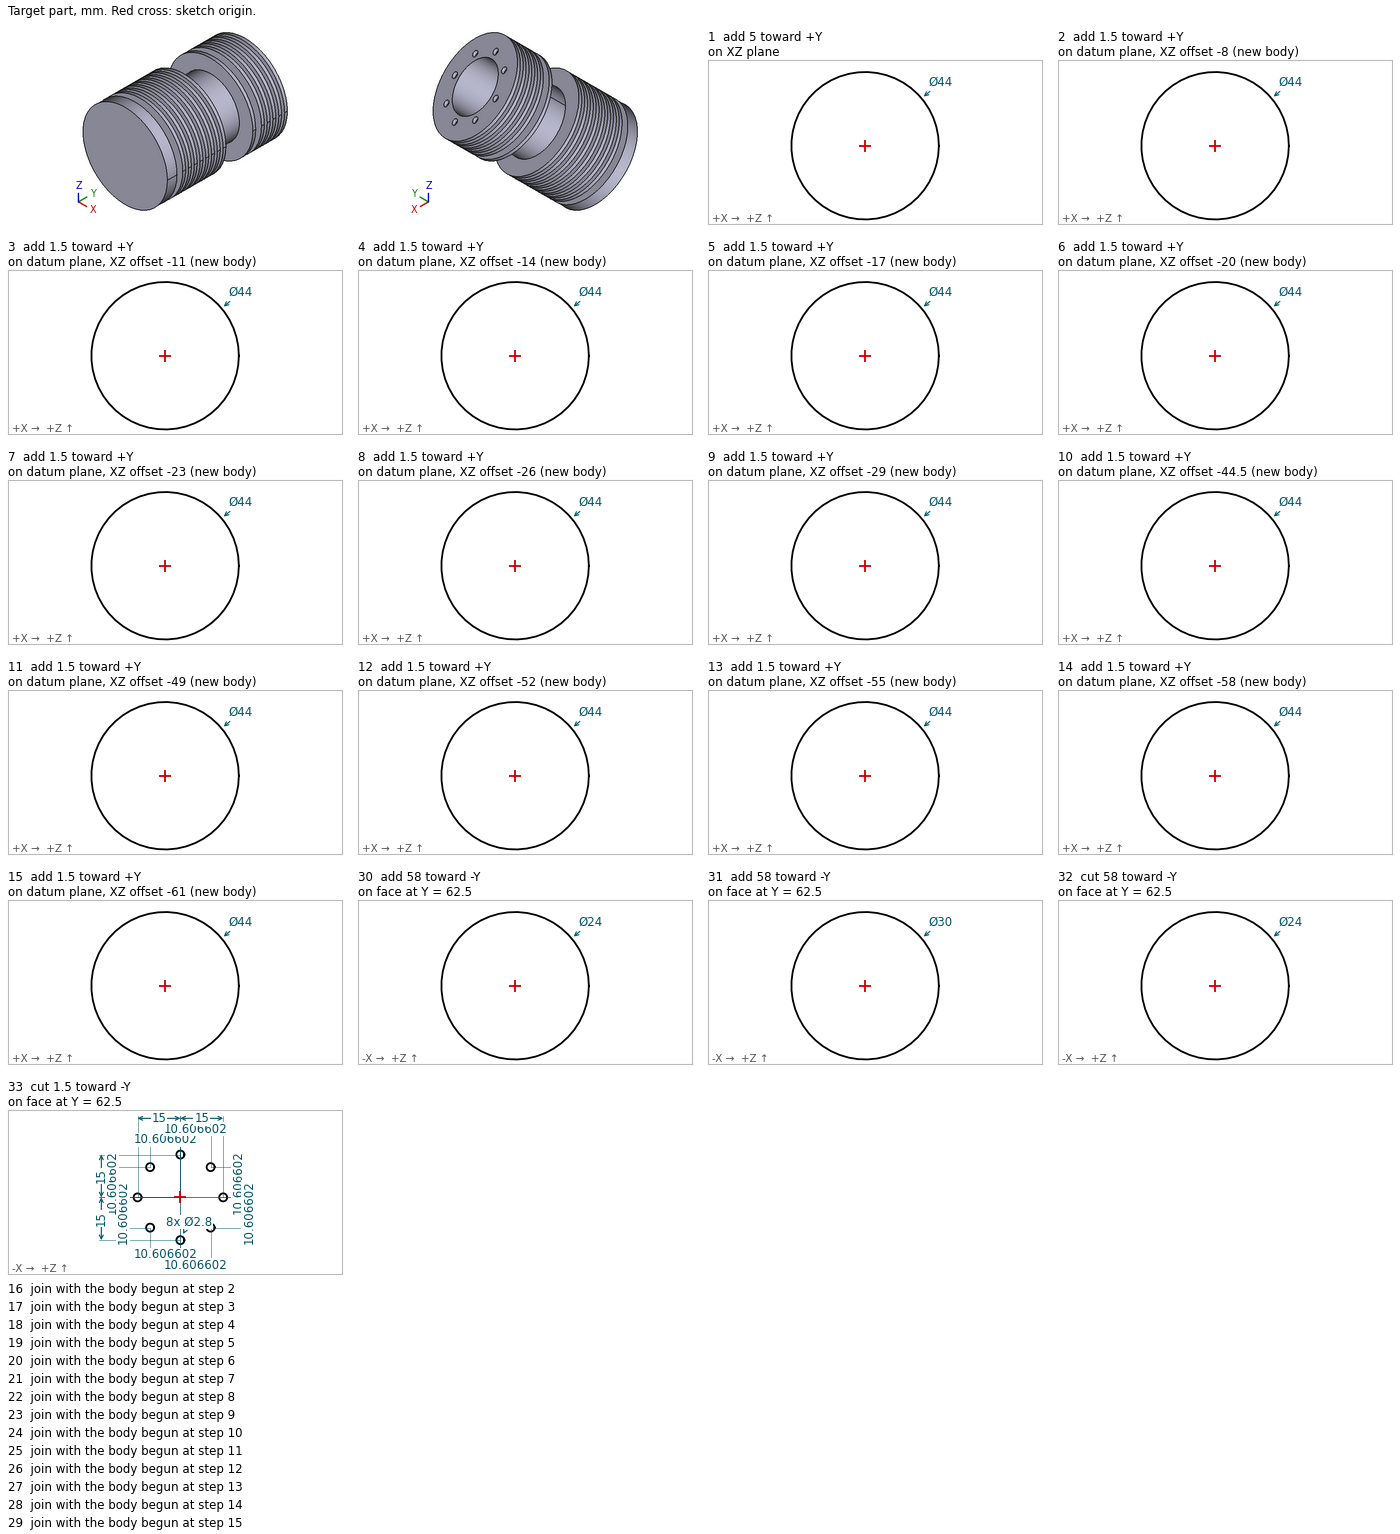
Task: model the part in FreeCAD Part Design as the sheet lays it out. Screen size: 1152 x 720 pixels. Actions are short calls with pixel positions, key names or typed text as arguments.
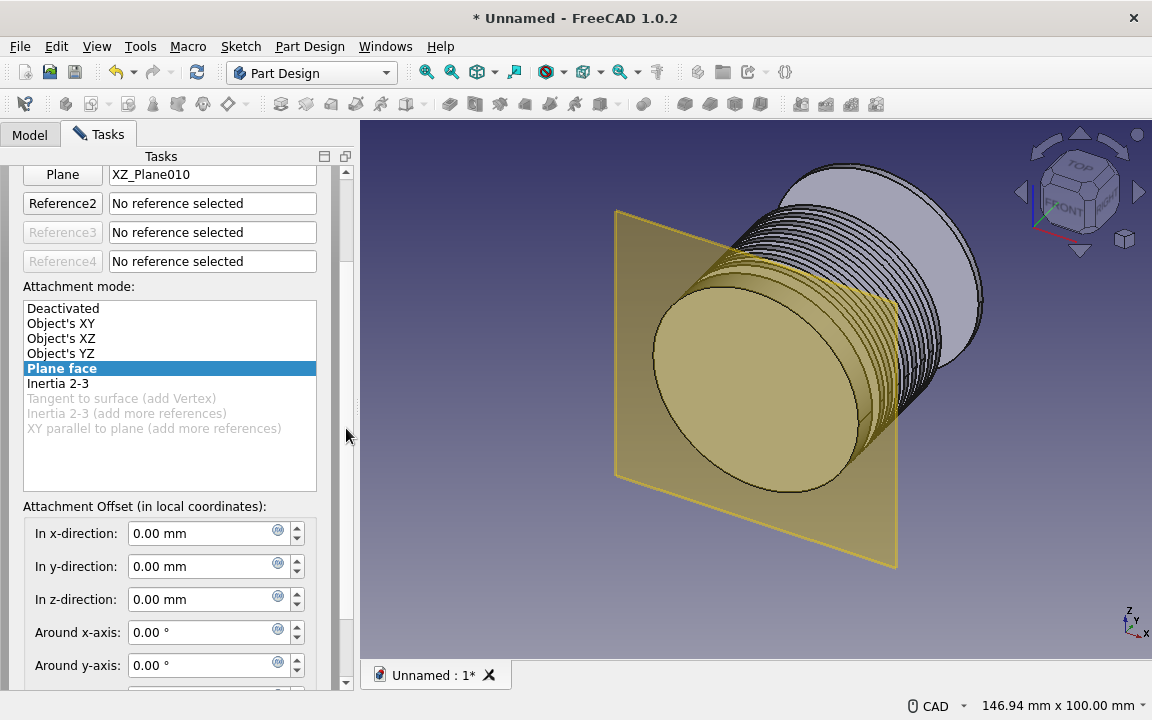
triple_click(210, 600)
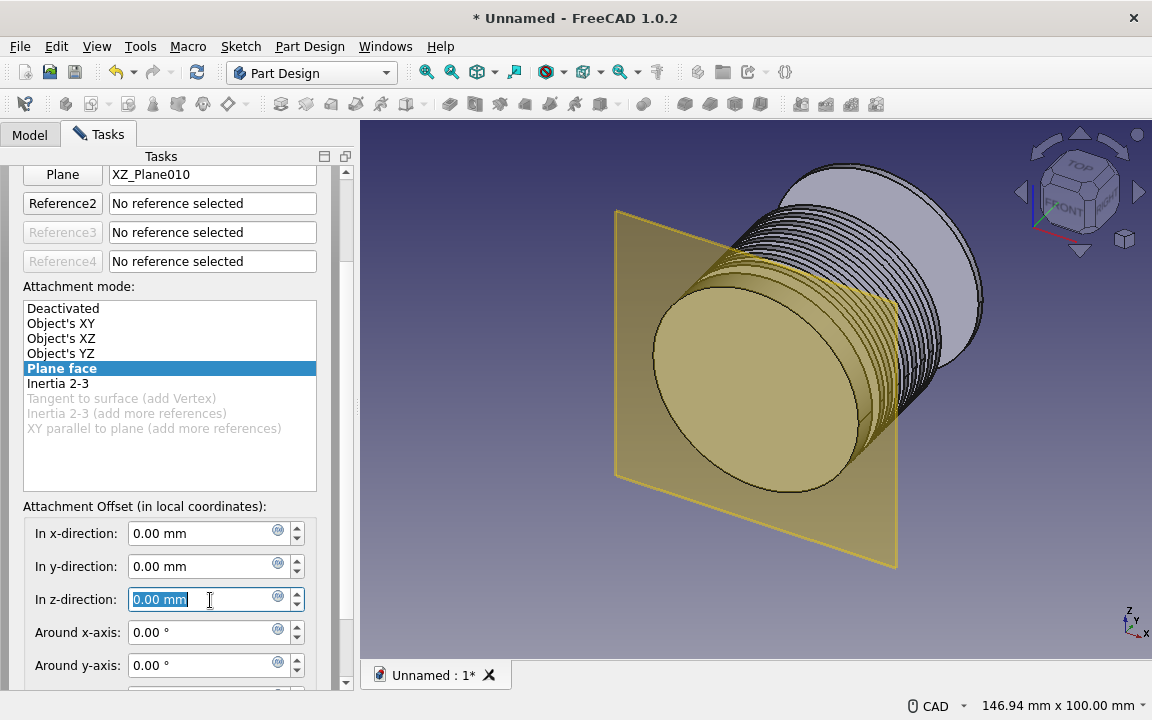
text(-49)
key(Tab)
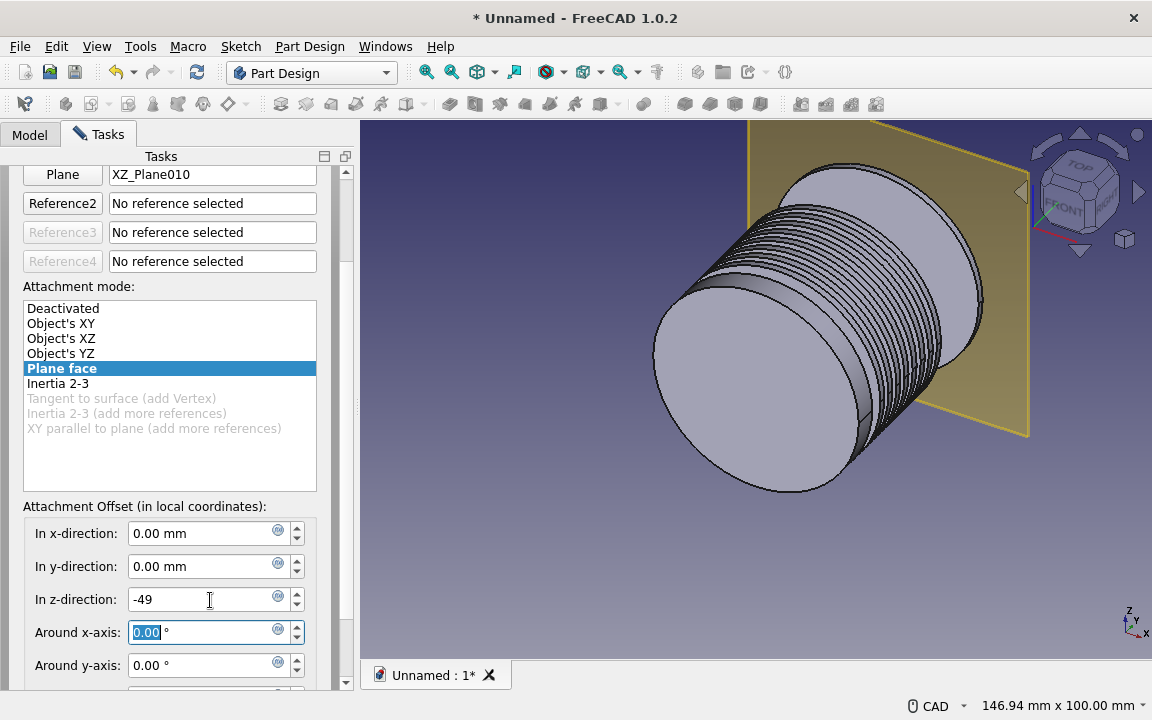
scroll(346, 428, up, 3)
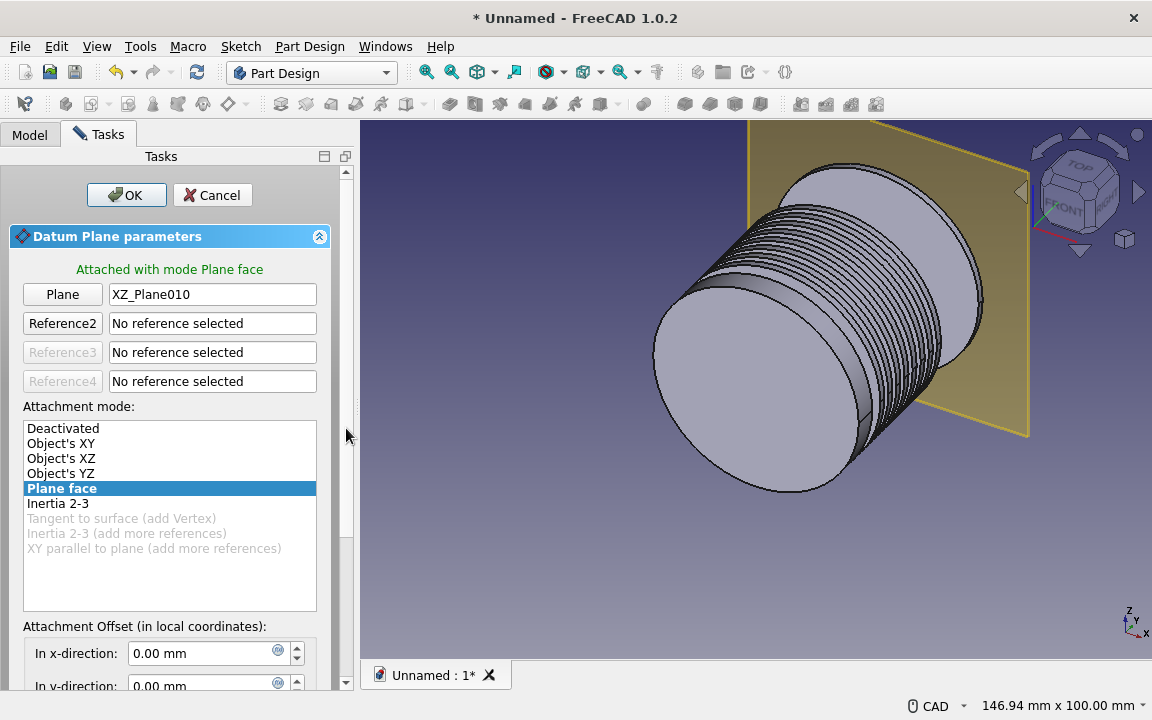
click(127, 195)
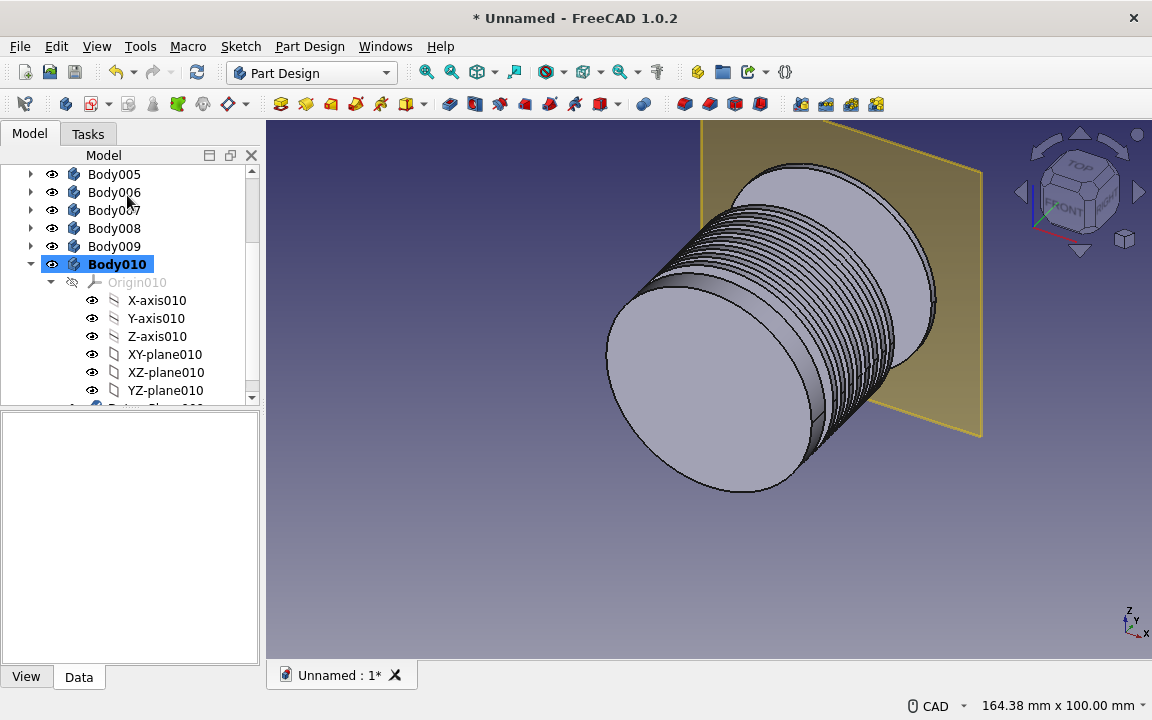
scroll(121, 278, down, 3)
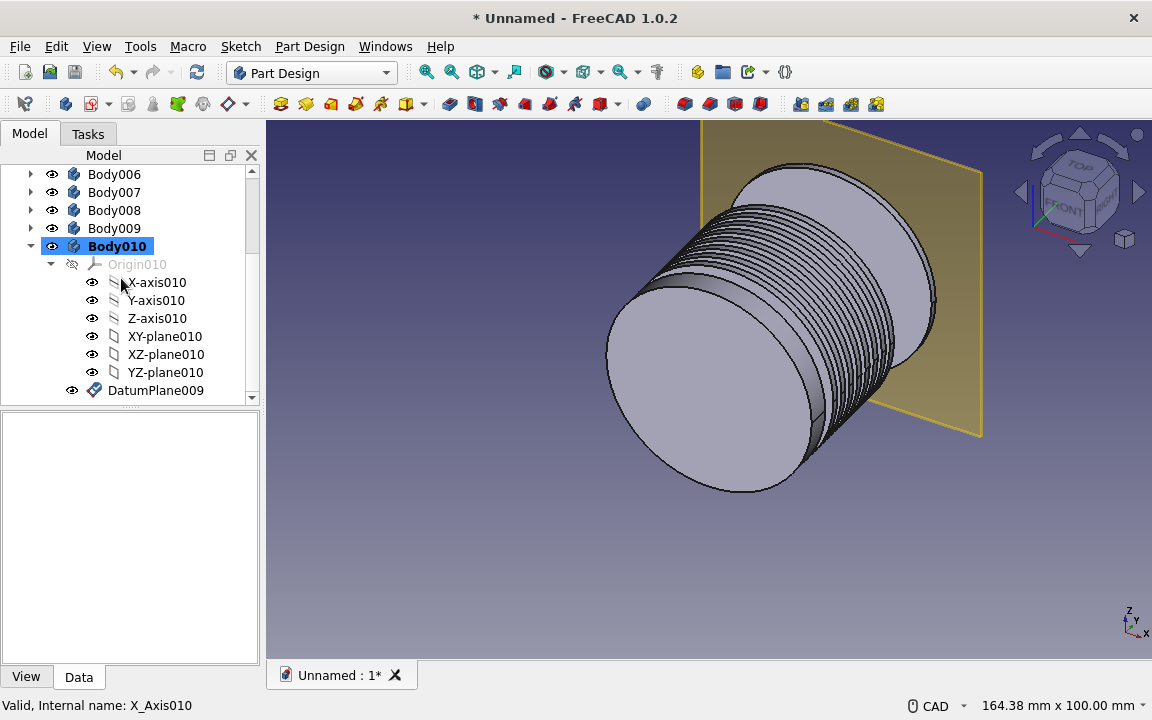
click(117, 390)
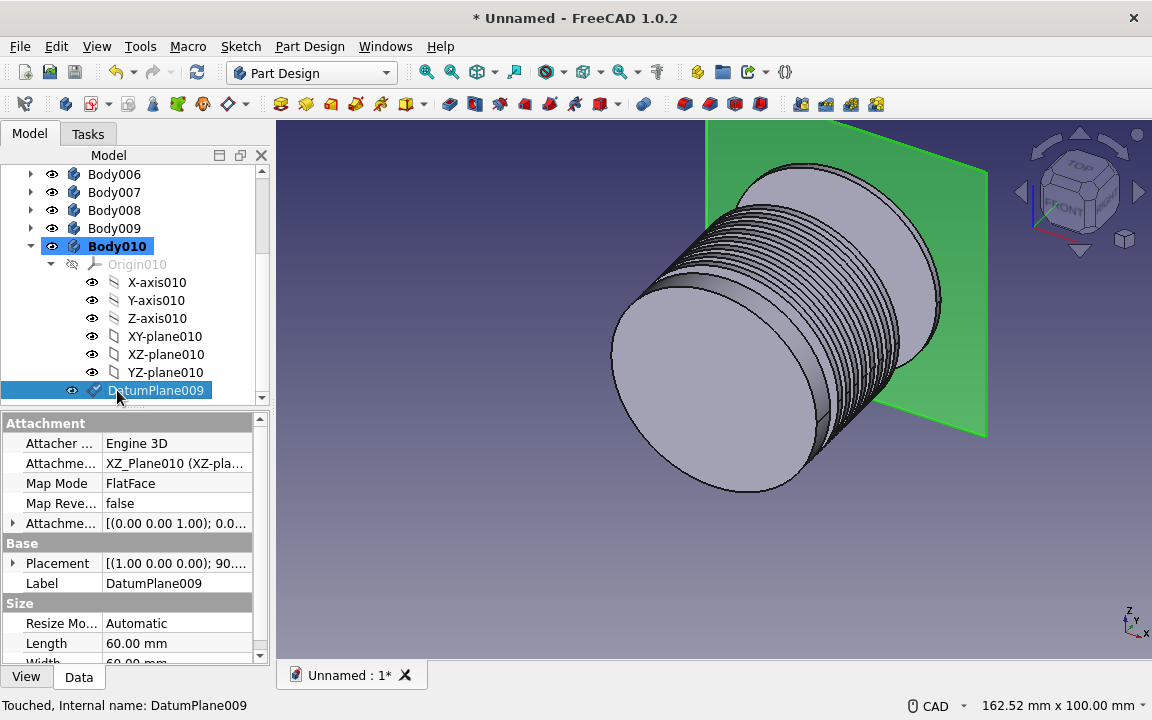
click(90, 104)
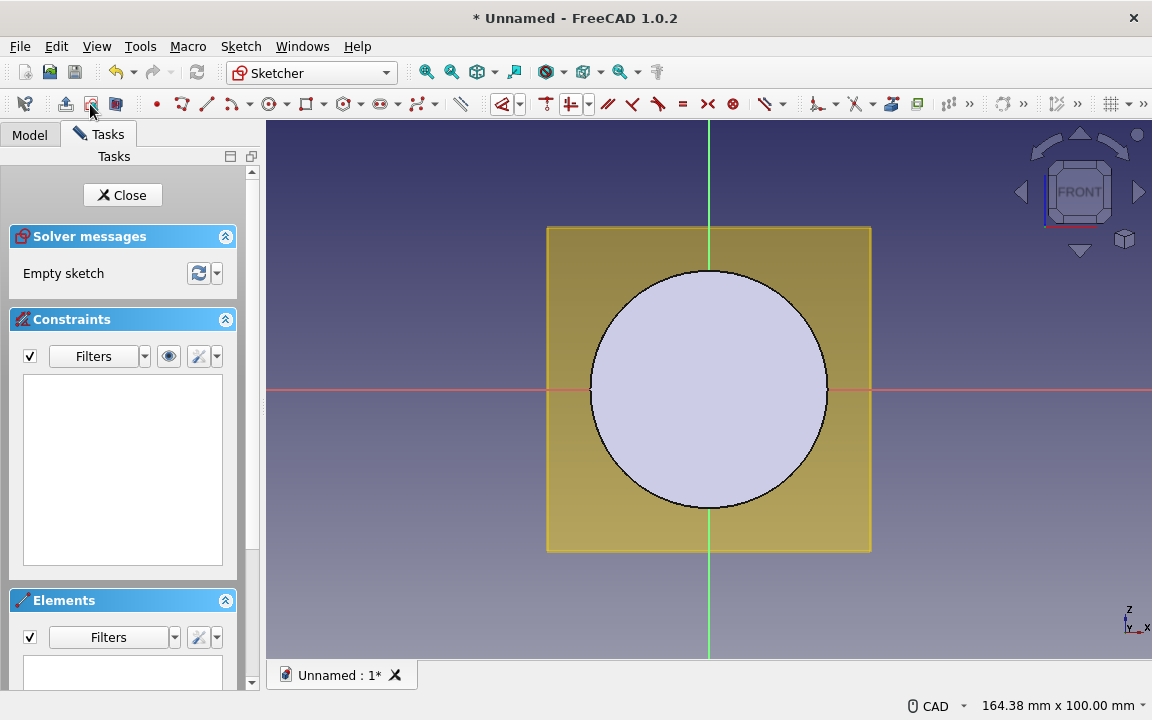
scroll(848, 390, up, 2)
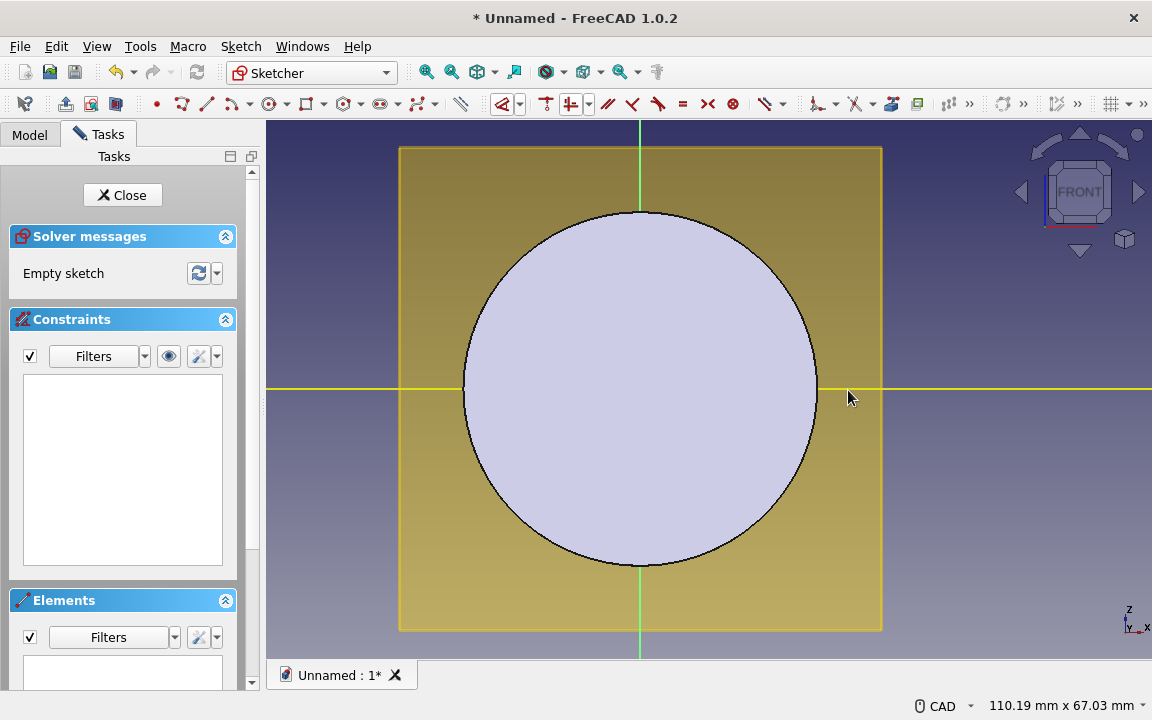
click(268, 104)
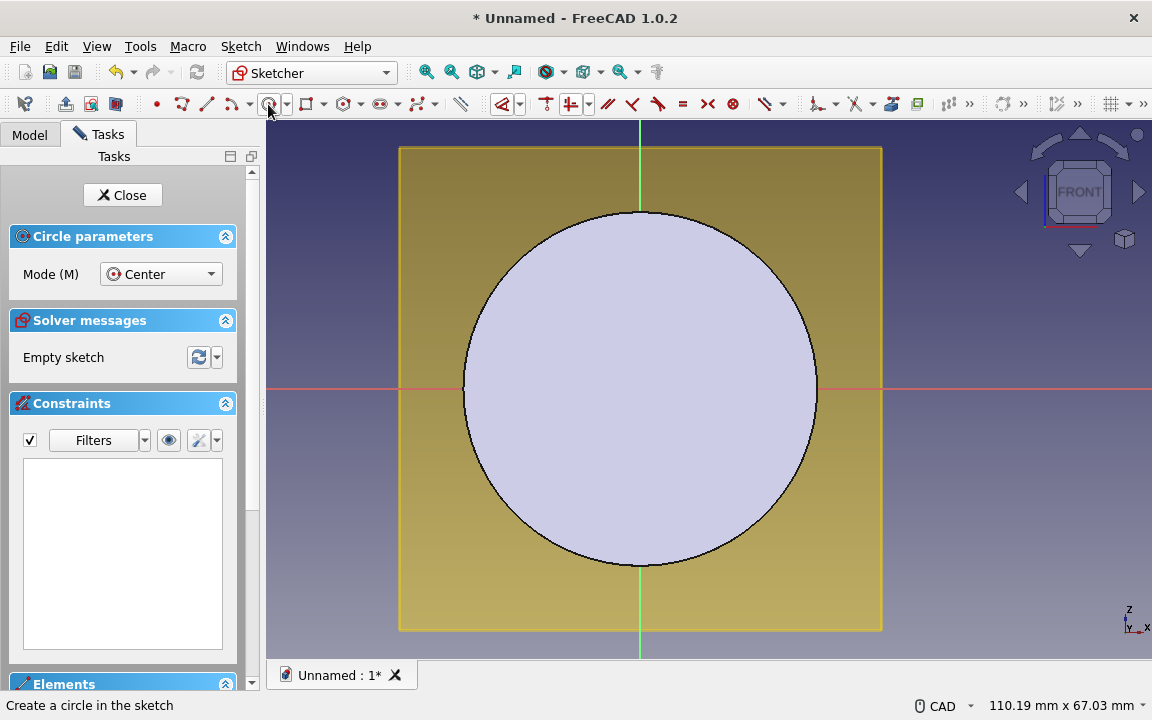
click(640, 389)
click(765, 264)
key(Escape)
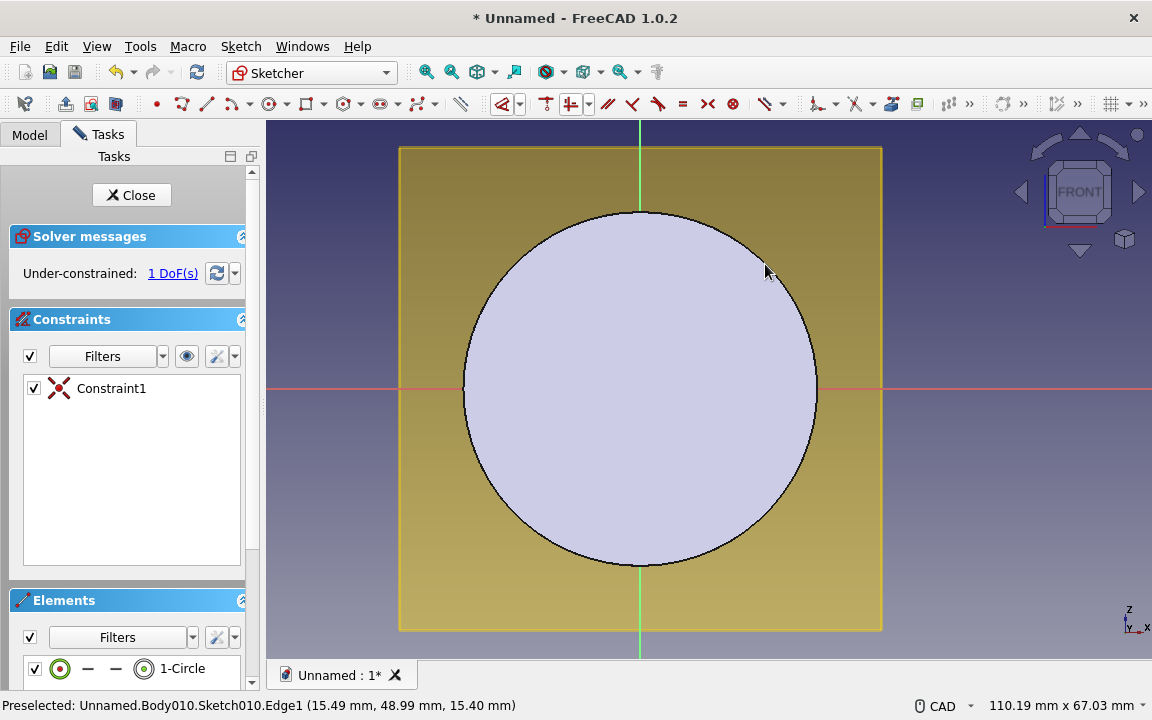
click(764, 264)